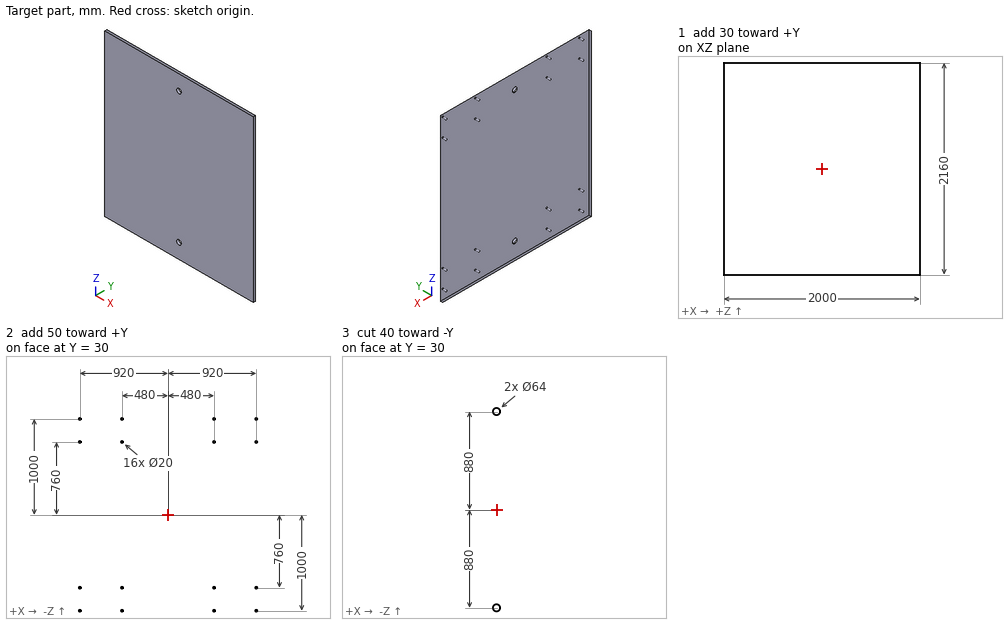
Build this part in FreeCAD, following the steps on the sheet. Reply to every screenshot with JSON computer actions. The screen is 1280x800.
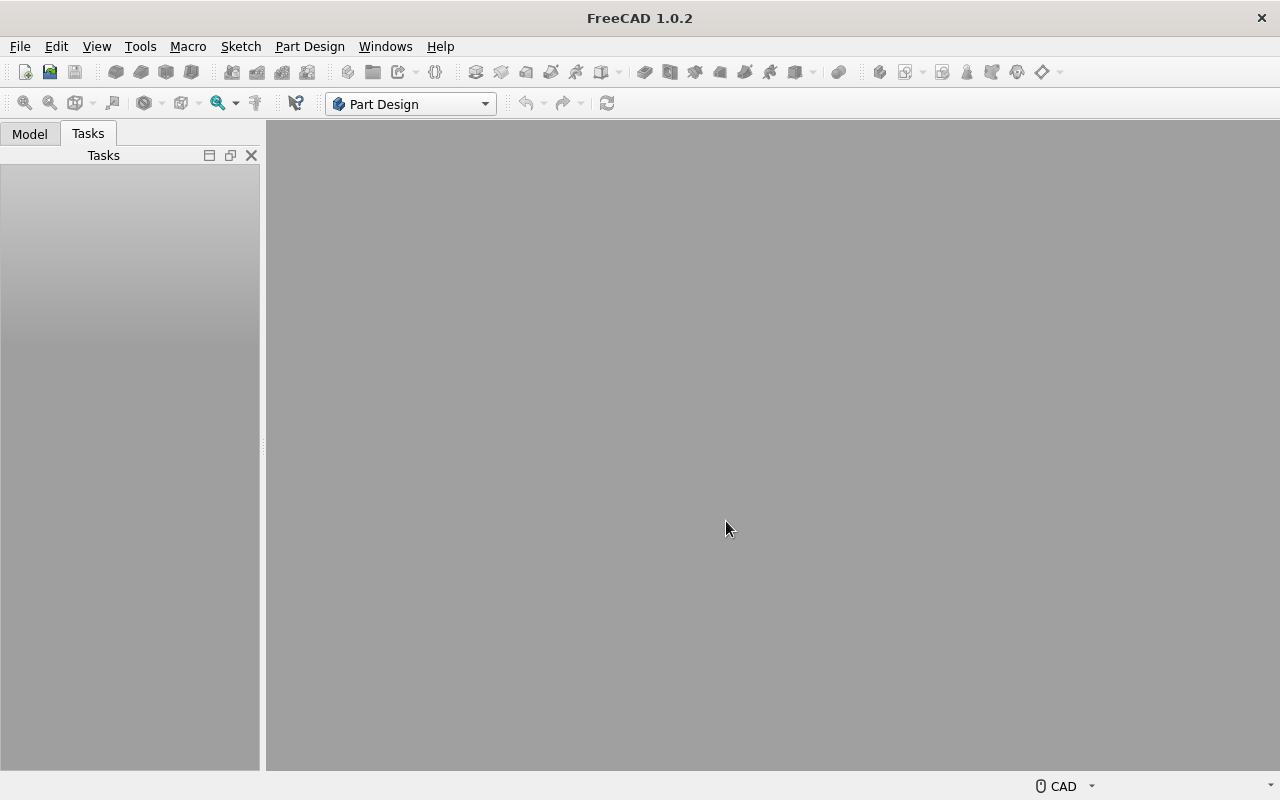
{"action": "left_click", "coordinate": [25, 72]}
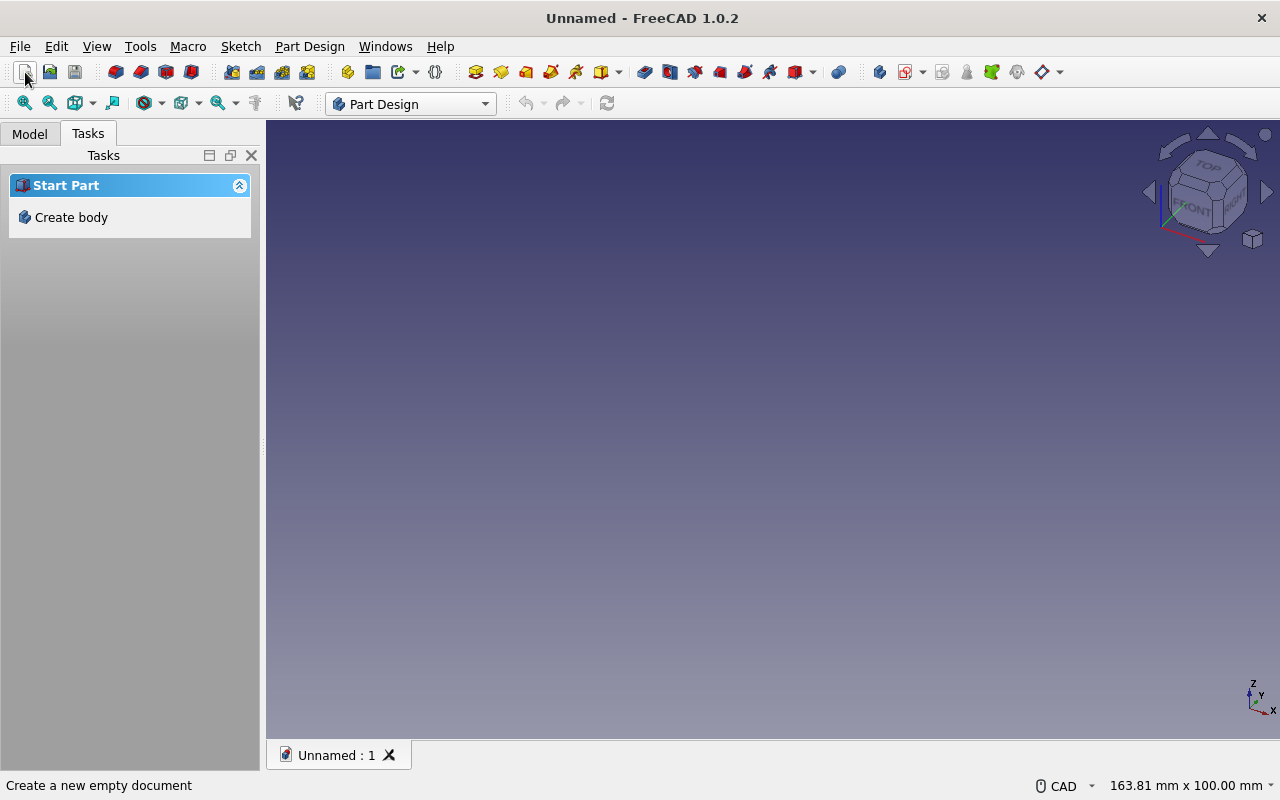
{"action": "left_click", "coordinate": [904, 72]}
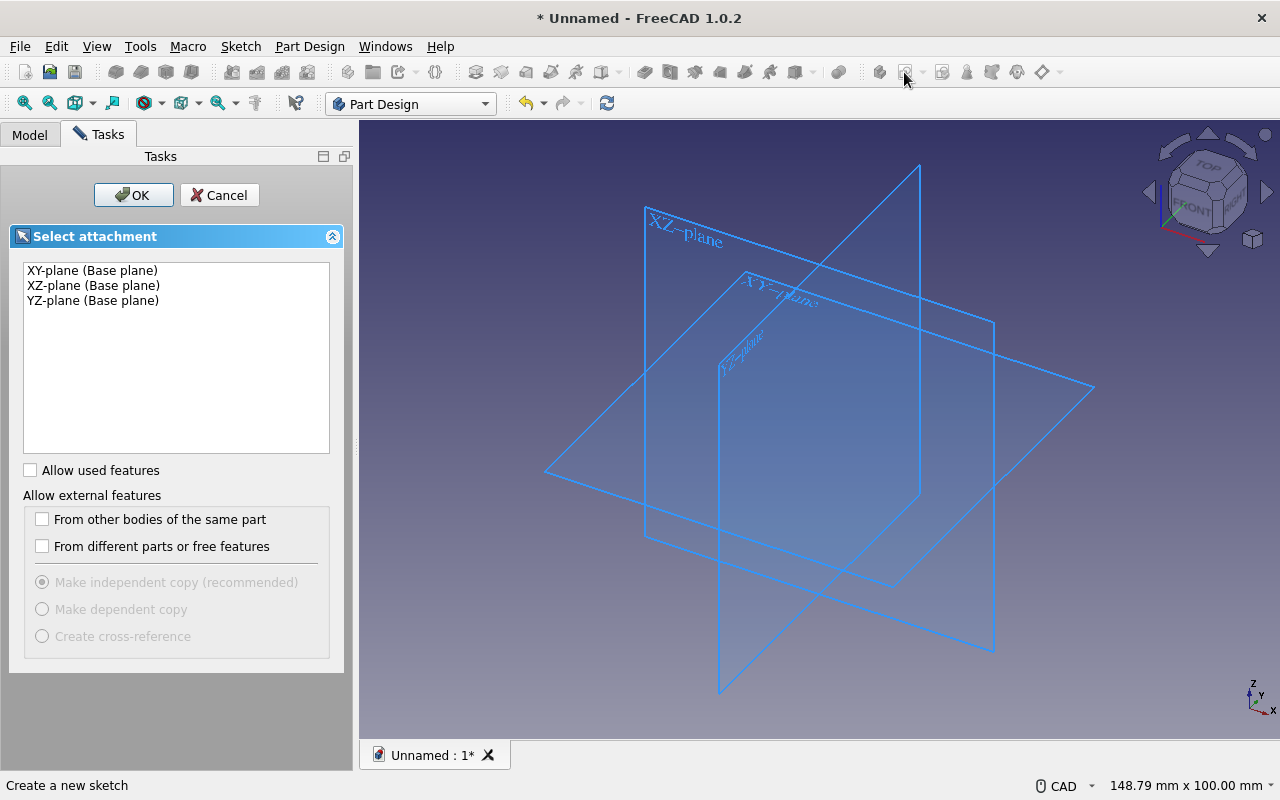
{"action": "left_click", "coordinate": [84, 286]}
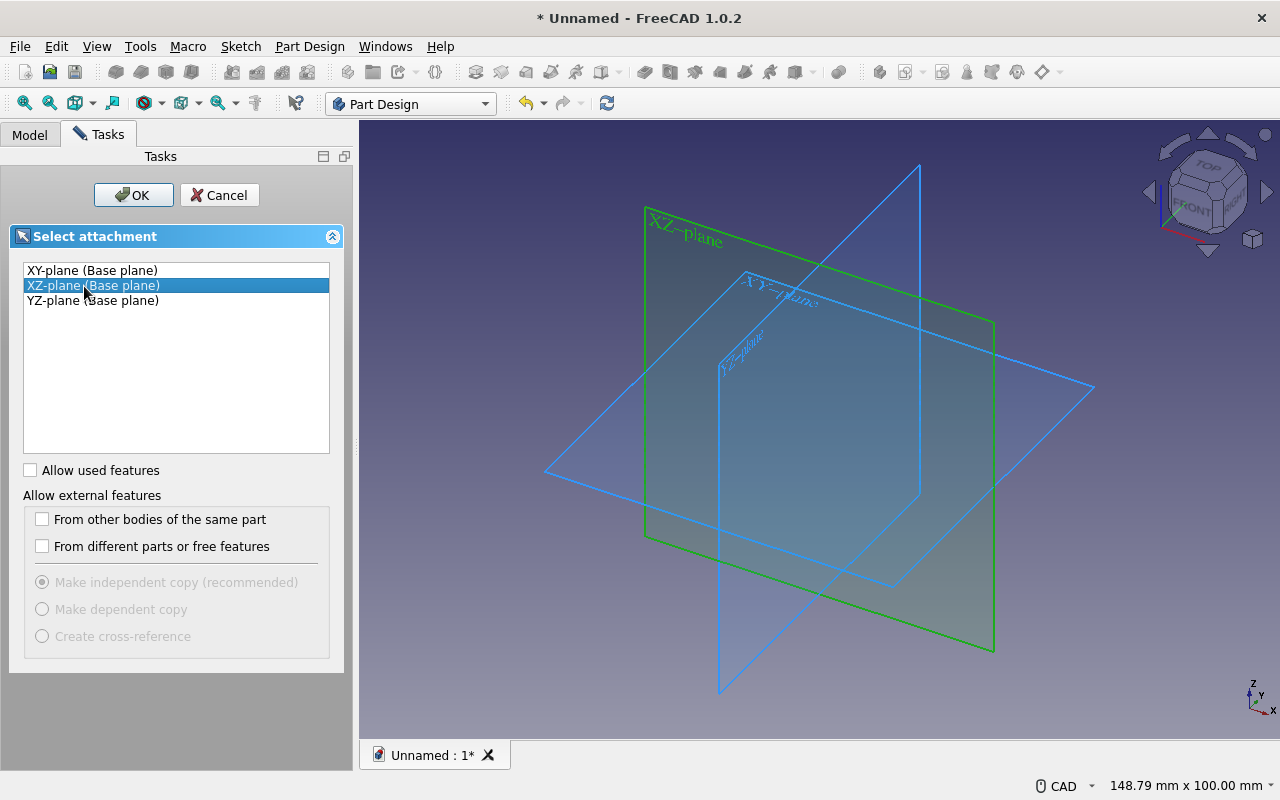
{"action": "left_click", "coordinate": [134, 195]}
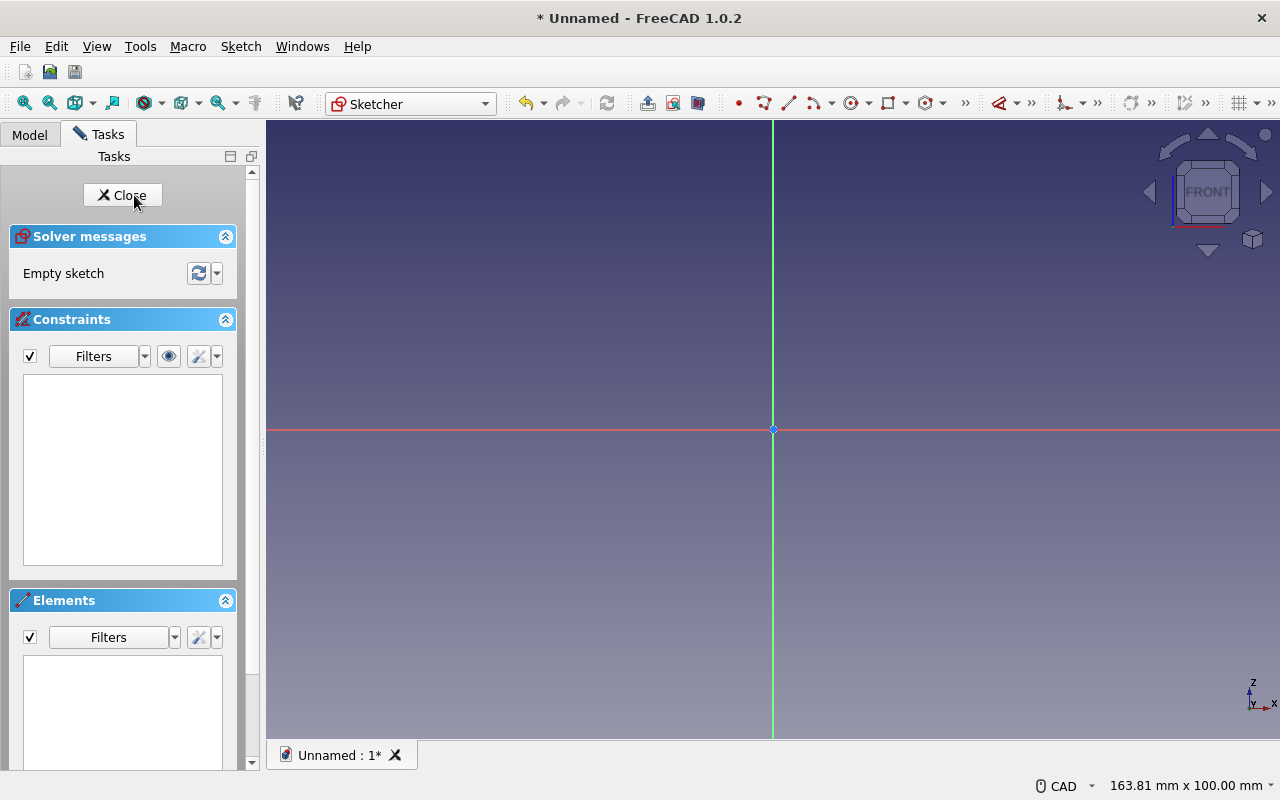
{"action": "scroll", "coordinate": [702, 430], "scroll_direction": "down", "scroll_amount": 17}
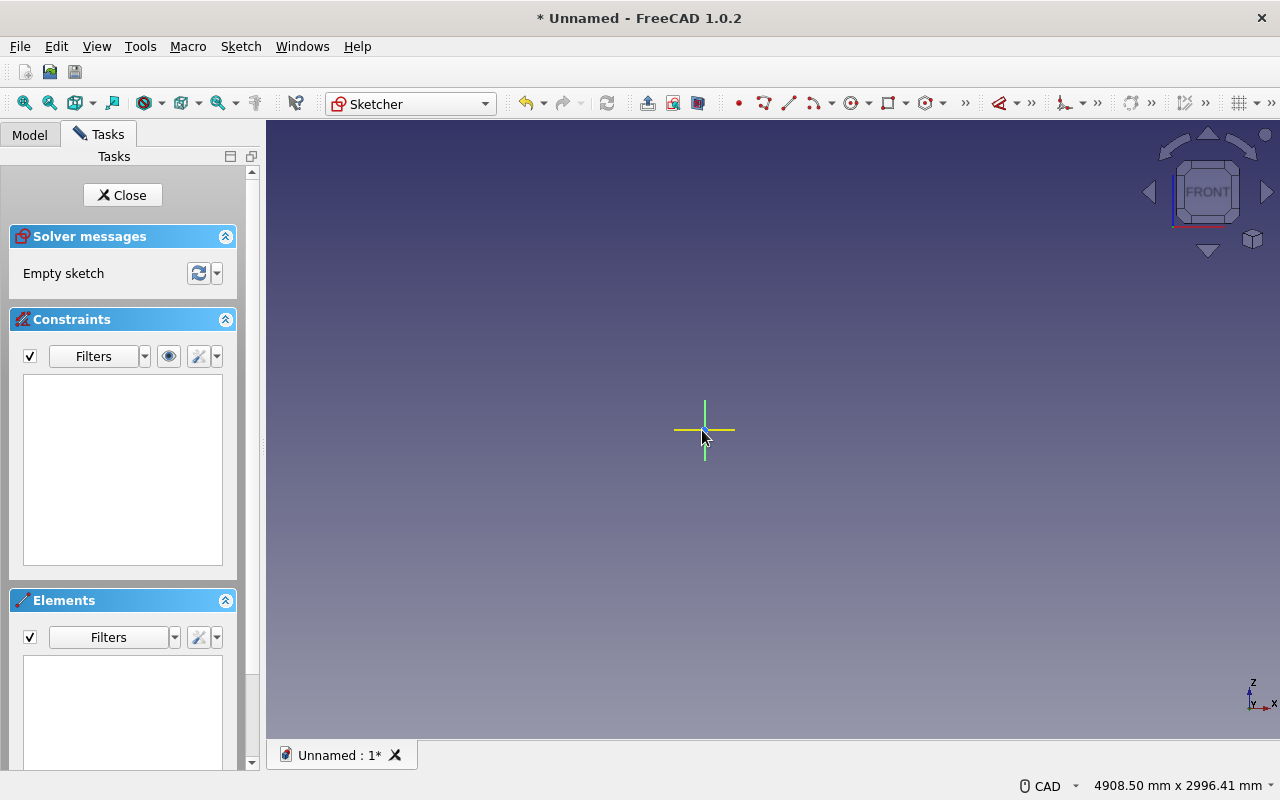
{"action": "left_click", "coordinate": [906, 104]}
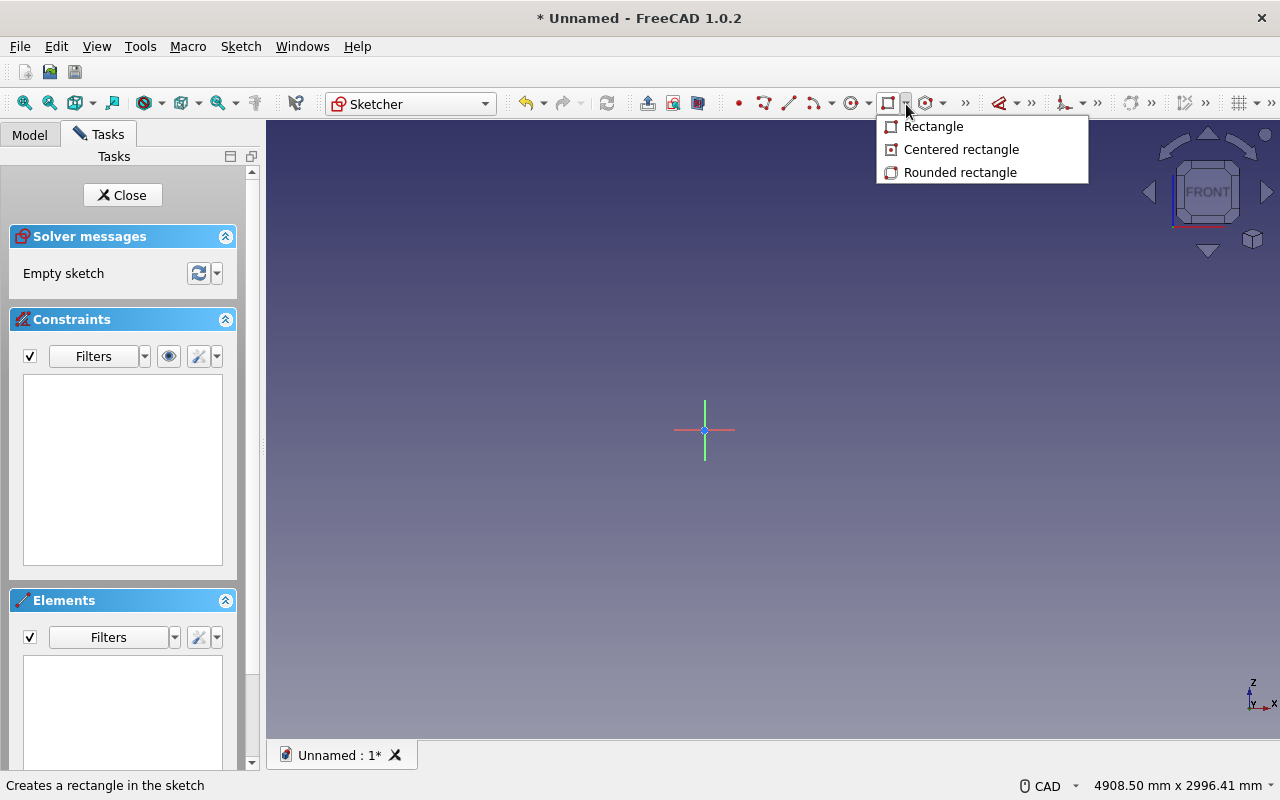
{"action": "left_click", "coordinate": [982, 150]}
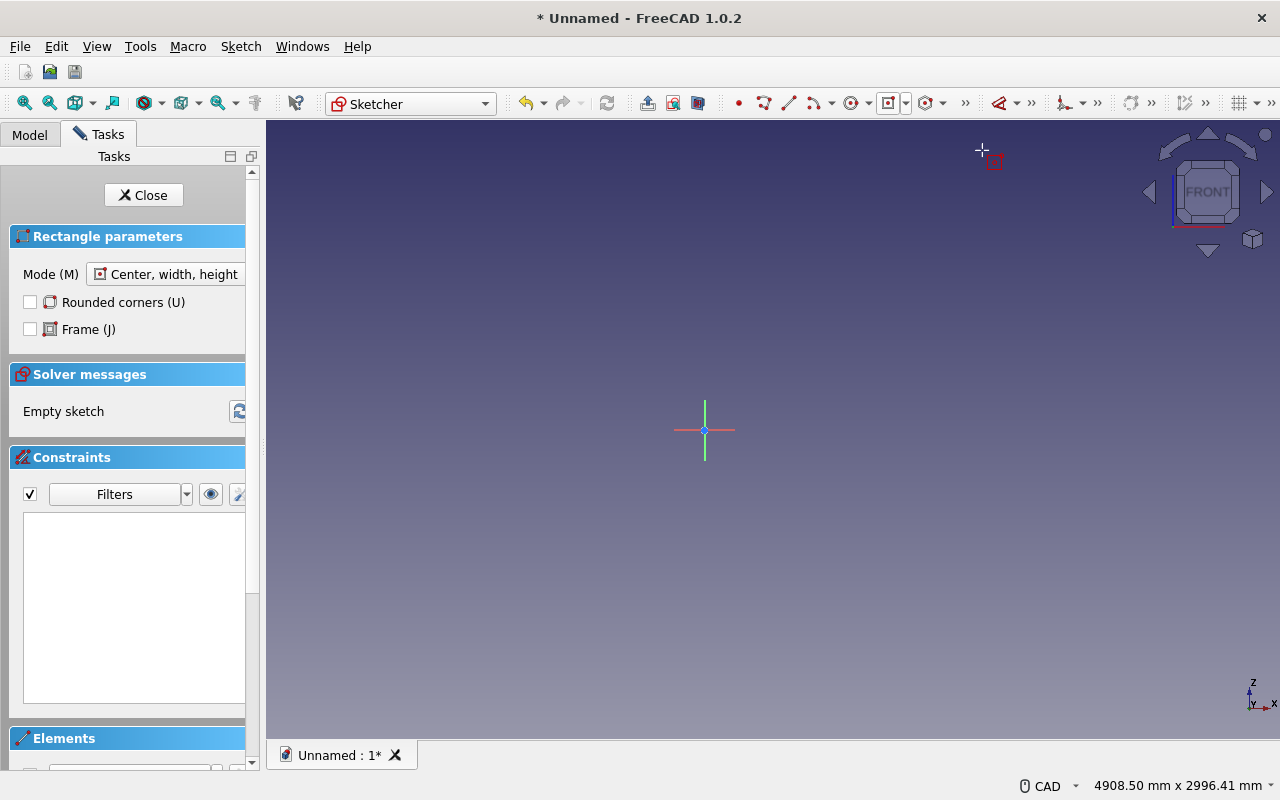
{"action": "left_click", "coordinate": [705, 430]}
{"action": "mouse_move", "coordinate": [911, 207]}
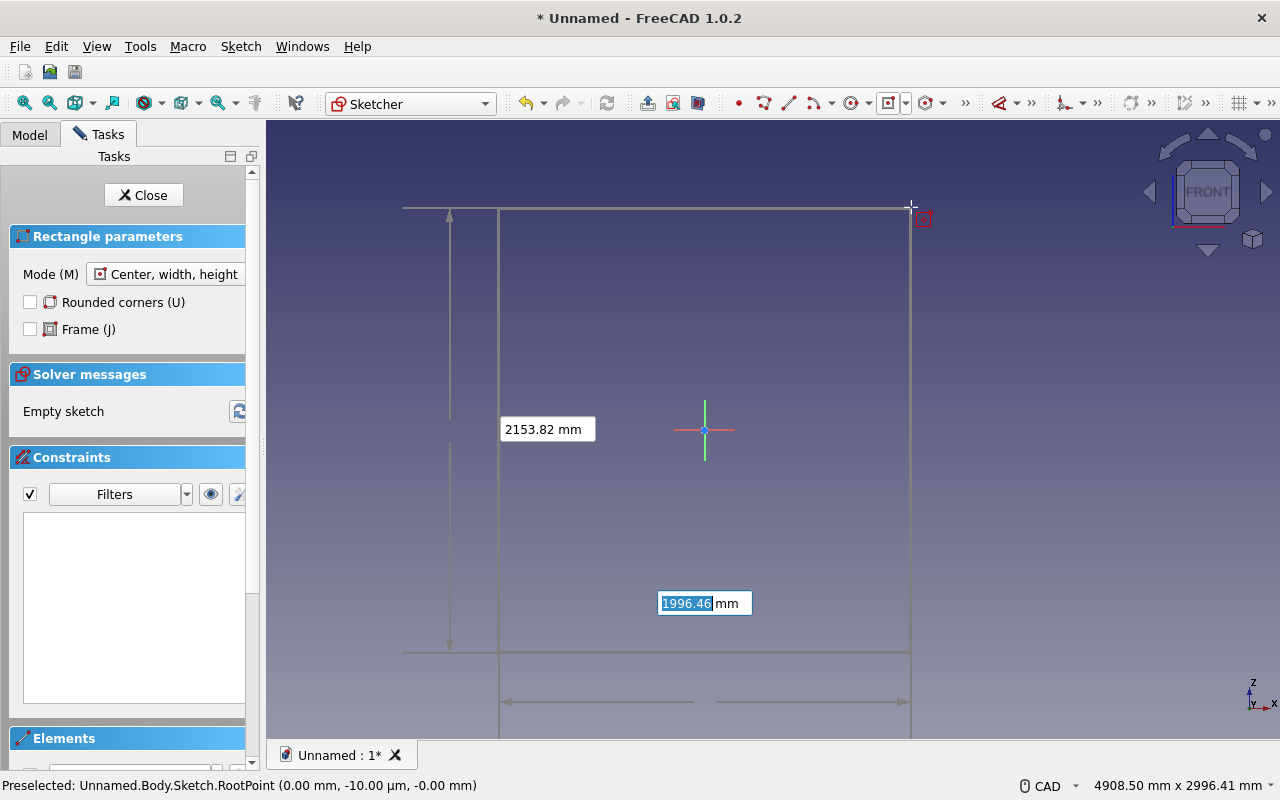
{"action": "type", "text": "2000"}
{"action": "key", "text": "Tab"}
{"action": "type", "text": "2160"}
{"action": "key", "text": "Return"}
{"action": "key", "text": "Escape"}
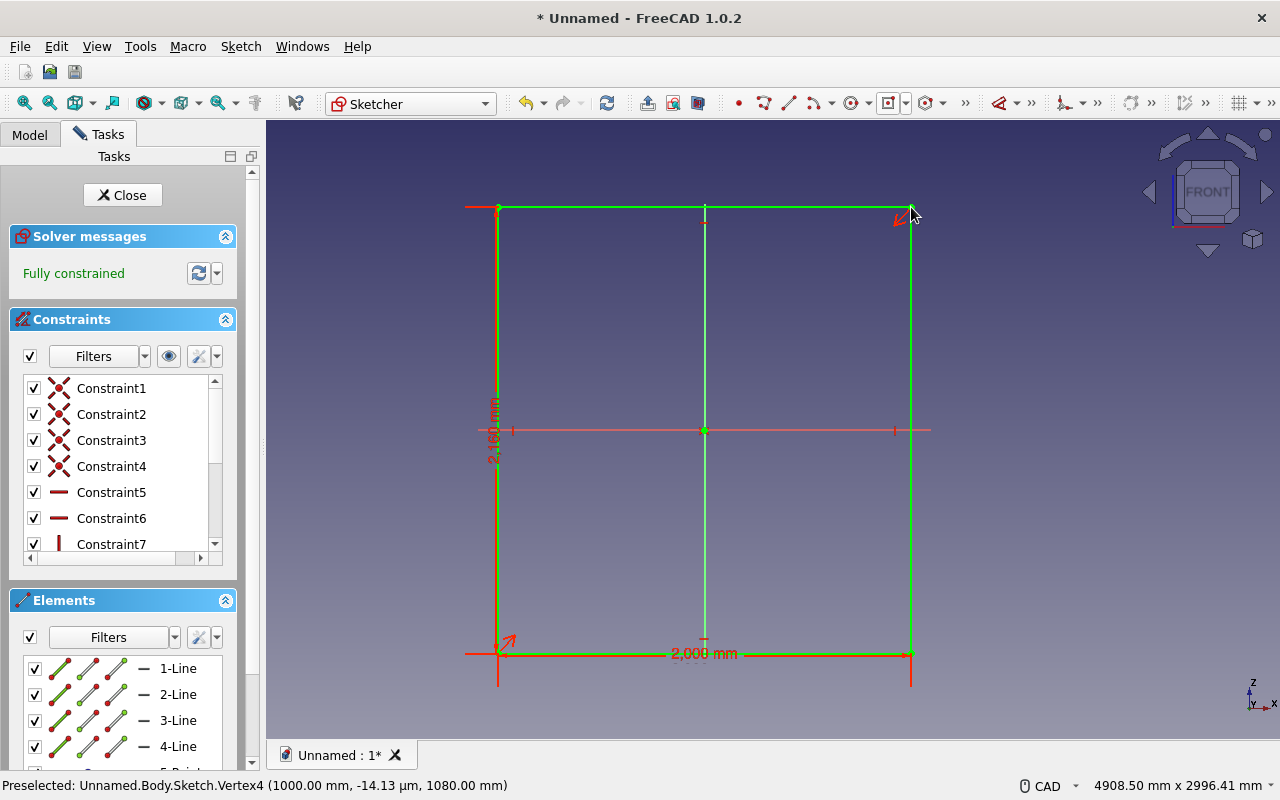
{"action": "left_click", "coordinate": [123, 195]}